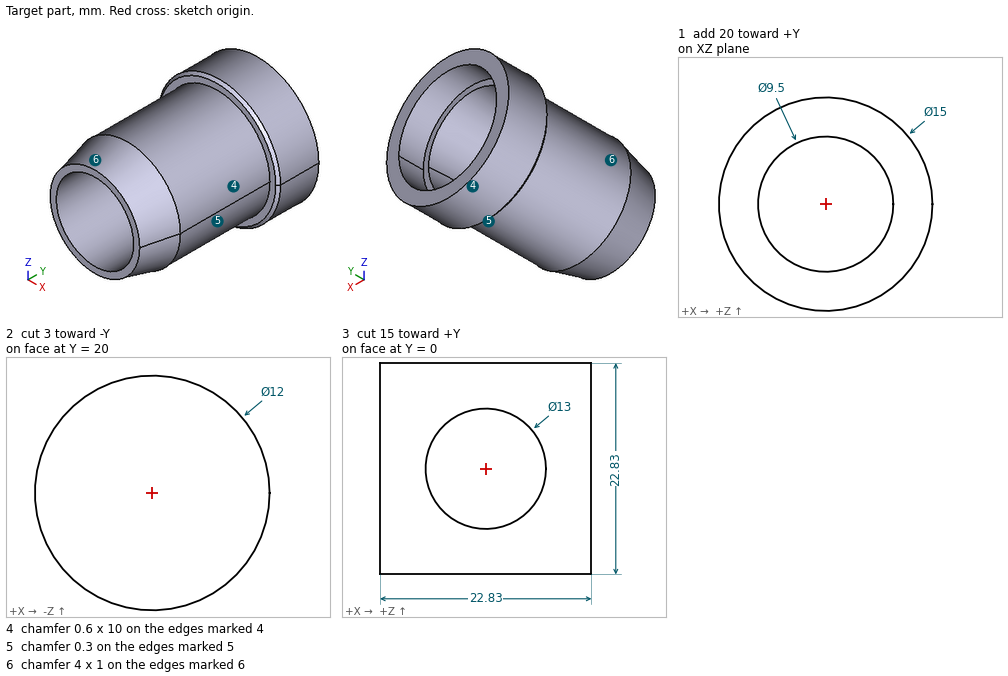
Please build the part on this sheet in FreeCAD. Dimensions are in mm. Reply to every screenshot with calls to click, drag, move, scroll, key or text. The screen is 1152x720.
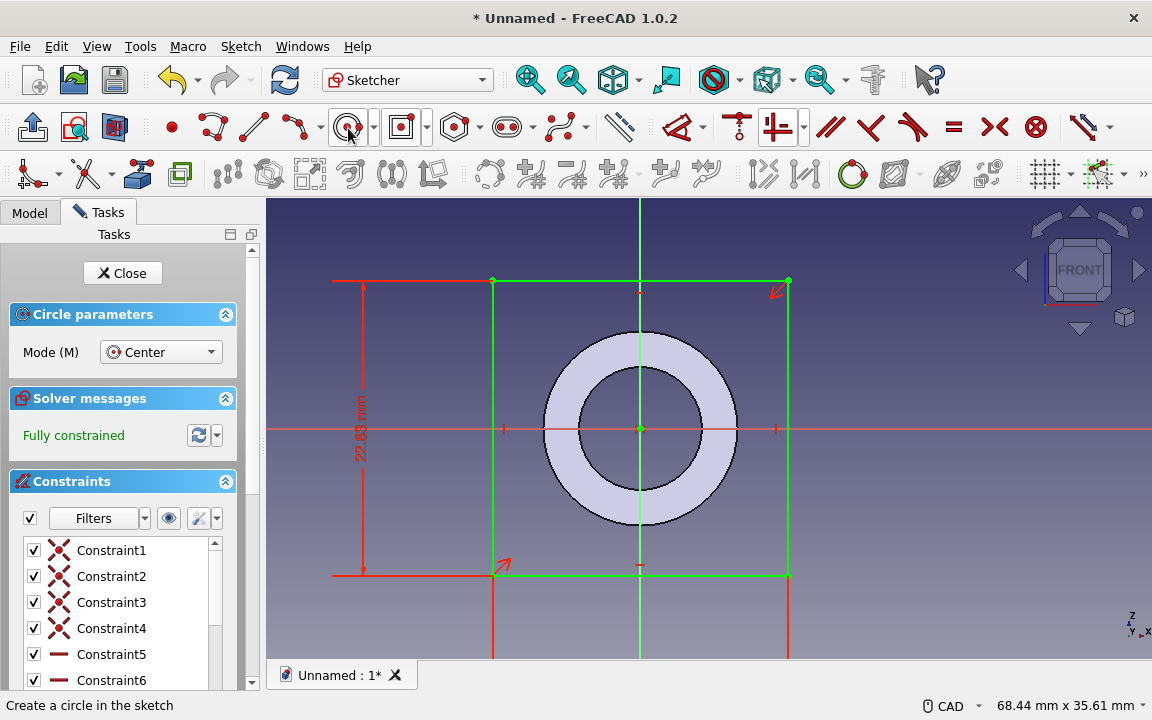
click(640, 429)
move(700, 369)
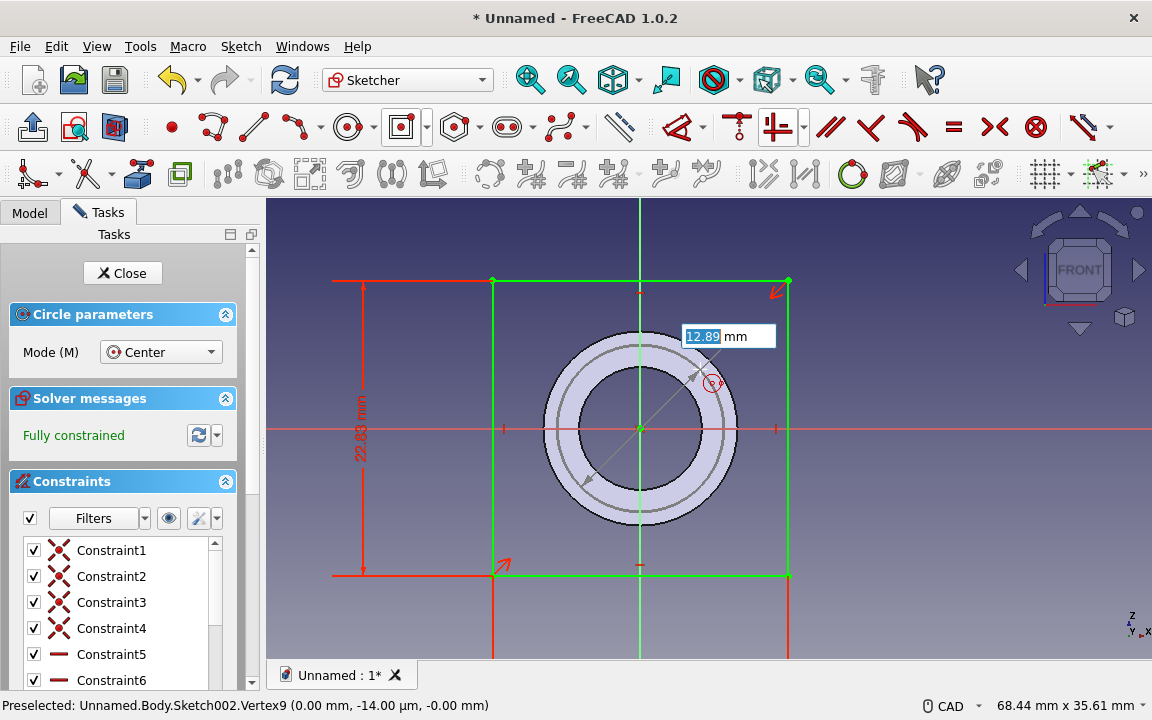
text(13)
key(Return)
key(Escape)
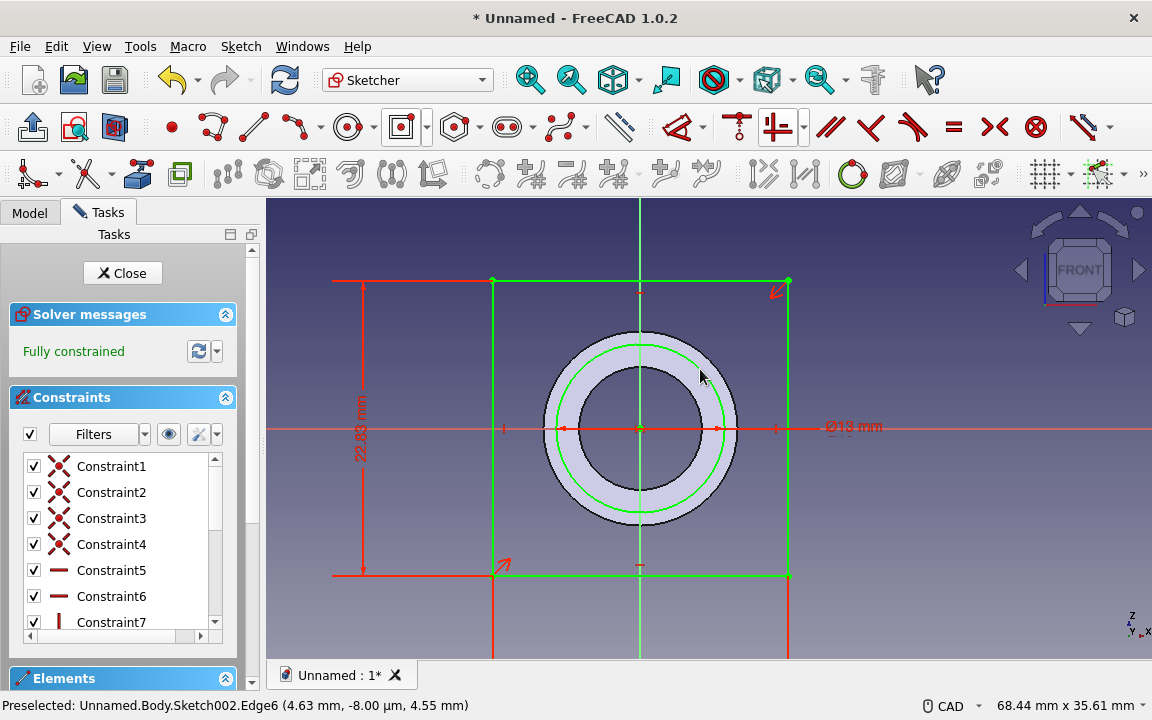
click(123, 273)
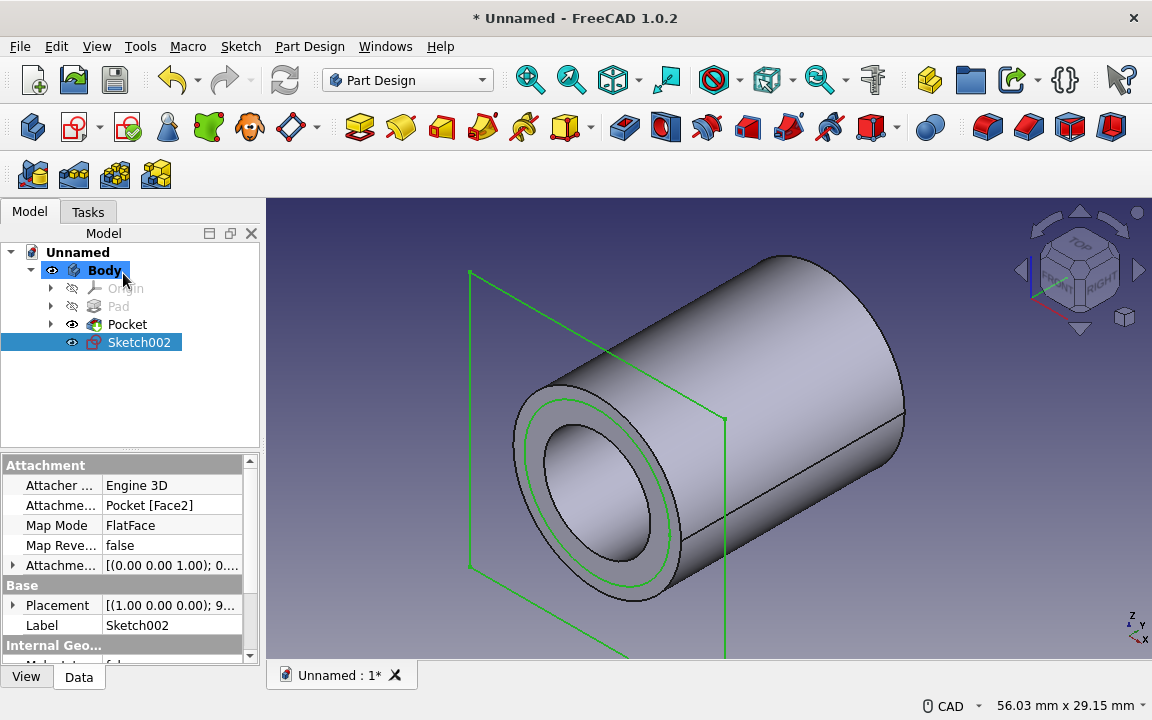
click(625, 128)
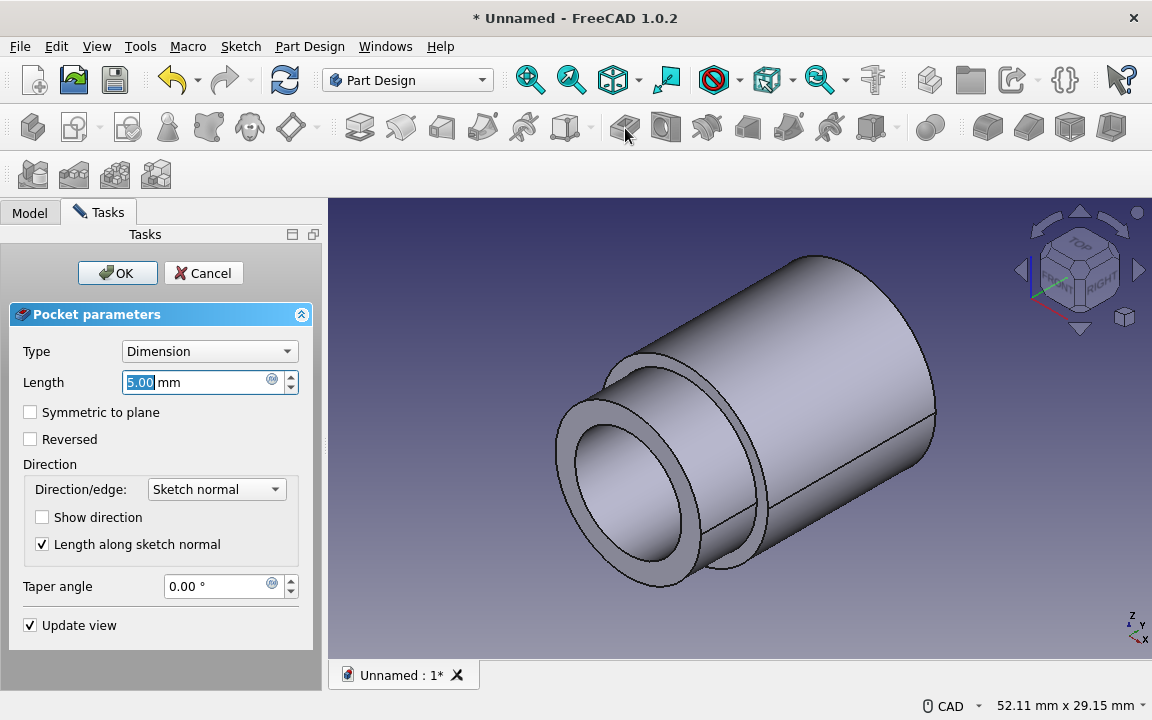
text(15)
key(Tab)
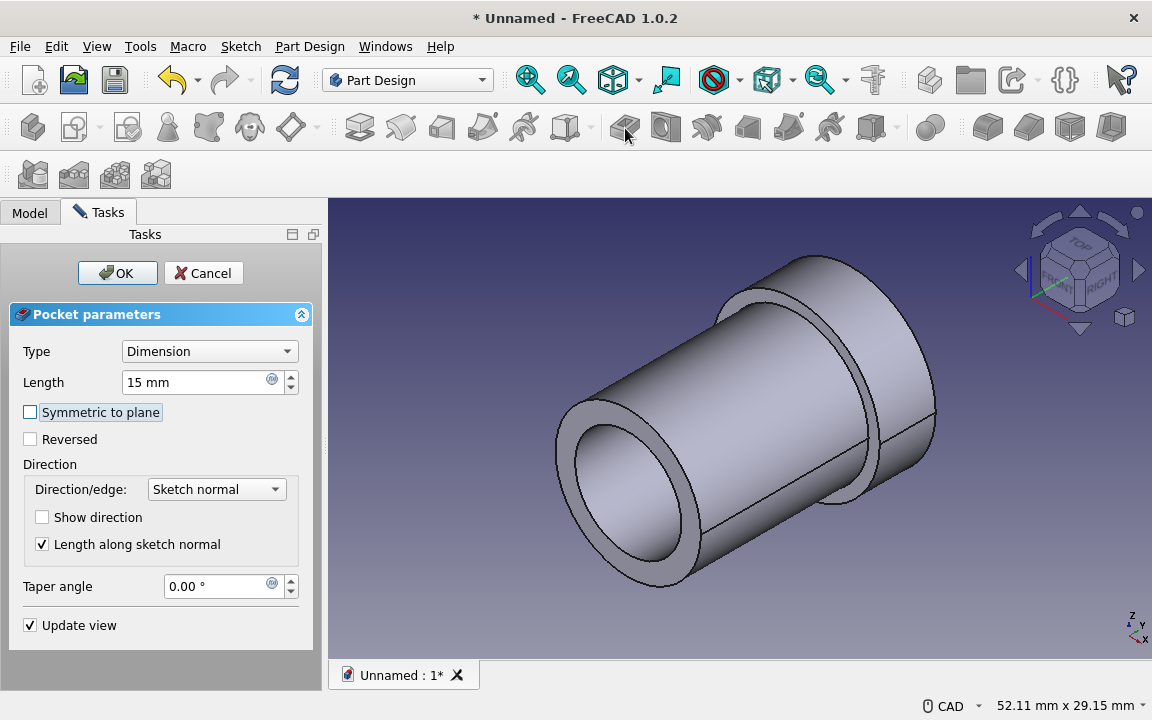
click(118, 273)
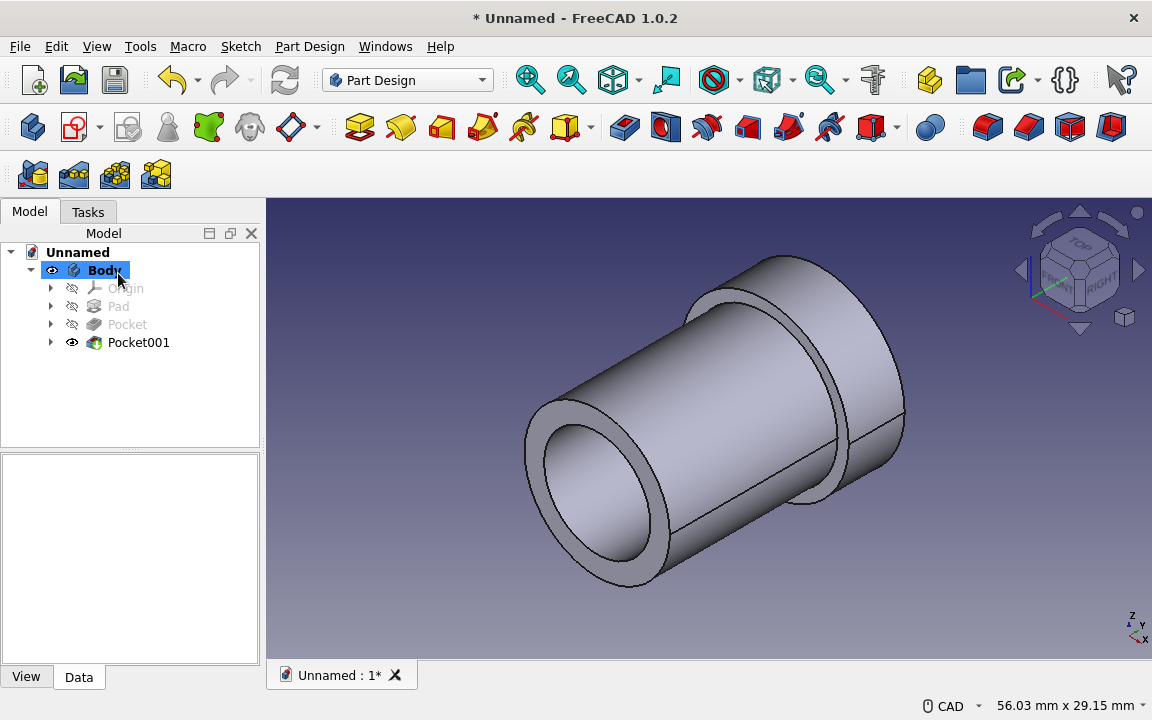
key(2)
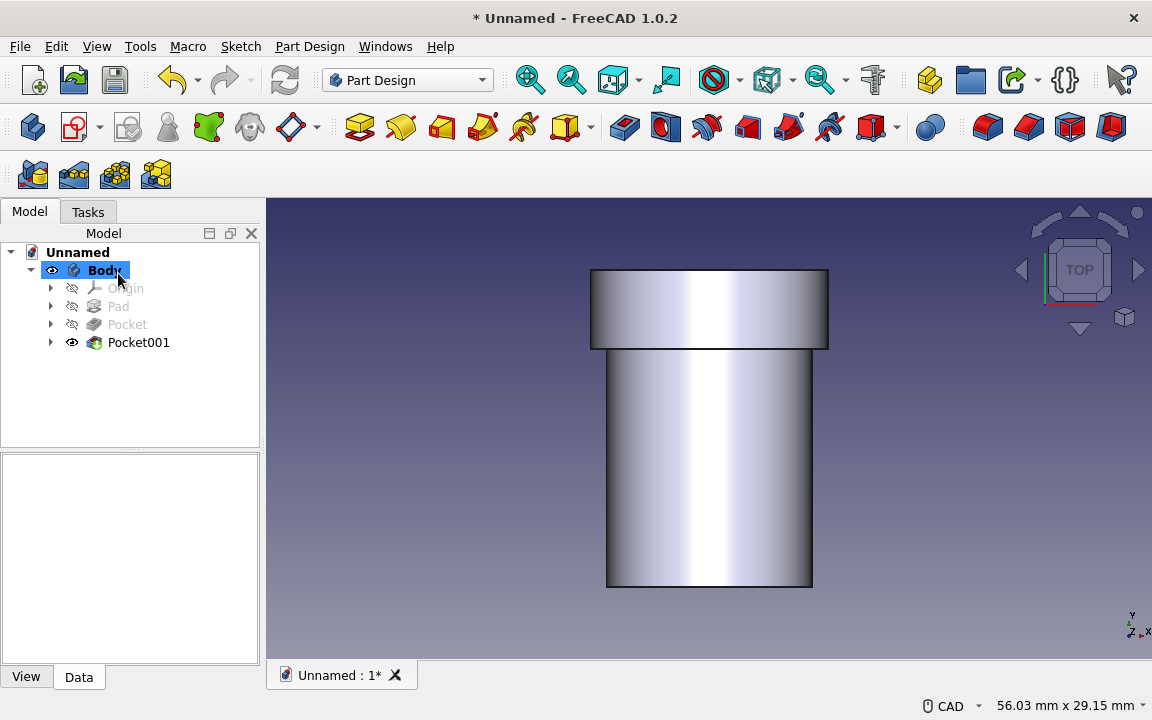
key(0)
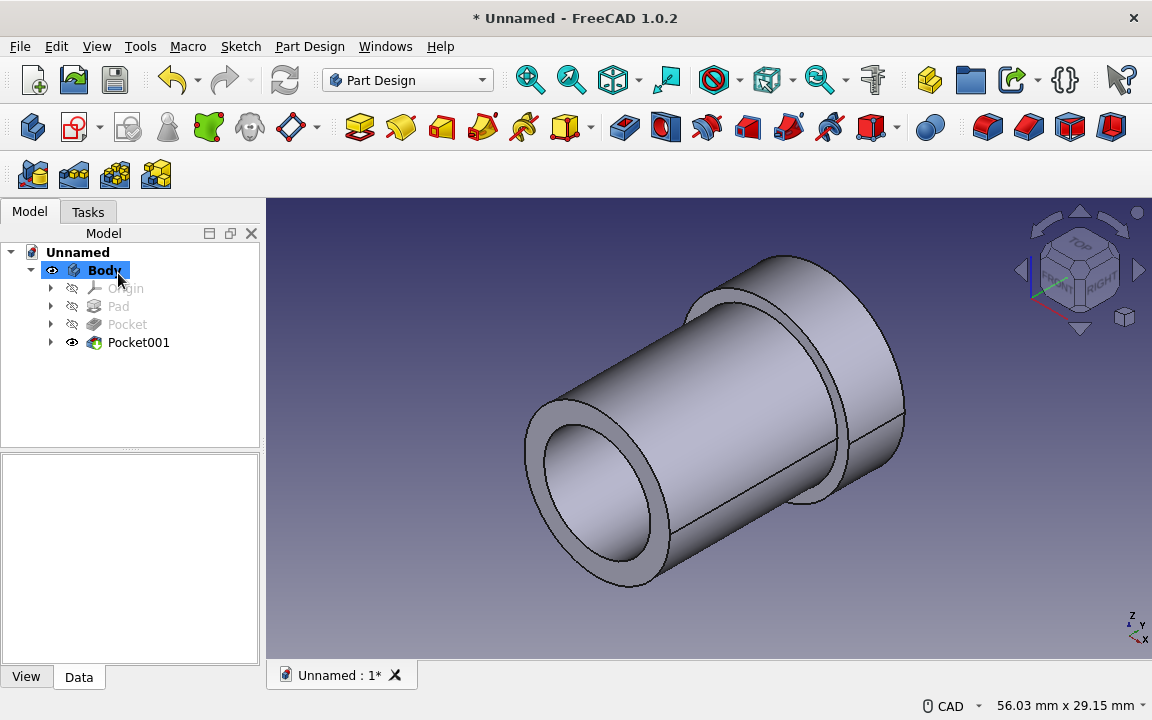
key(1)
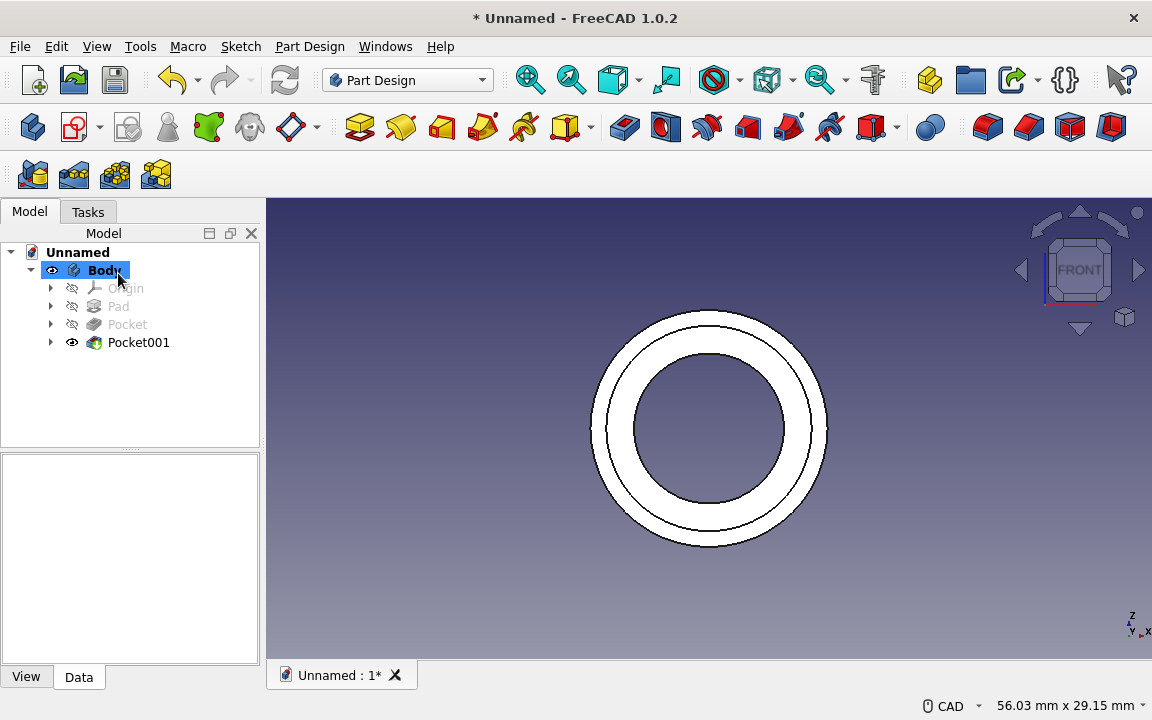
key(3)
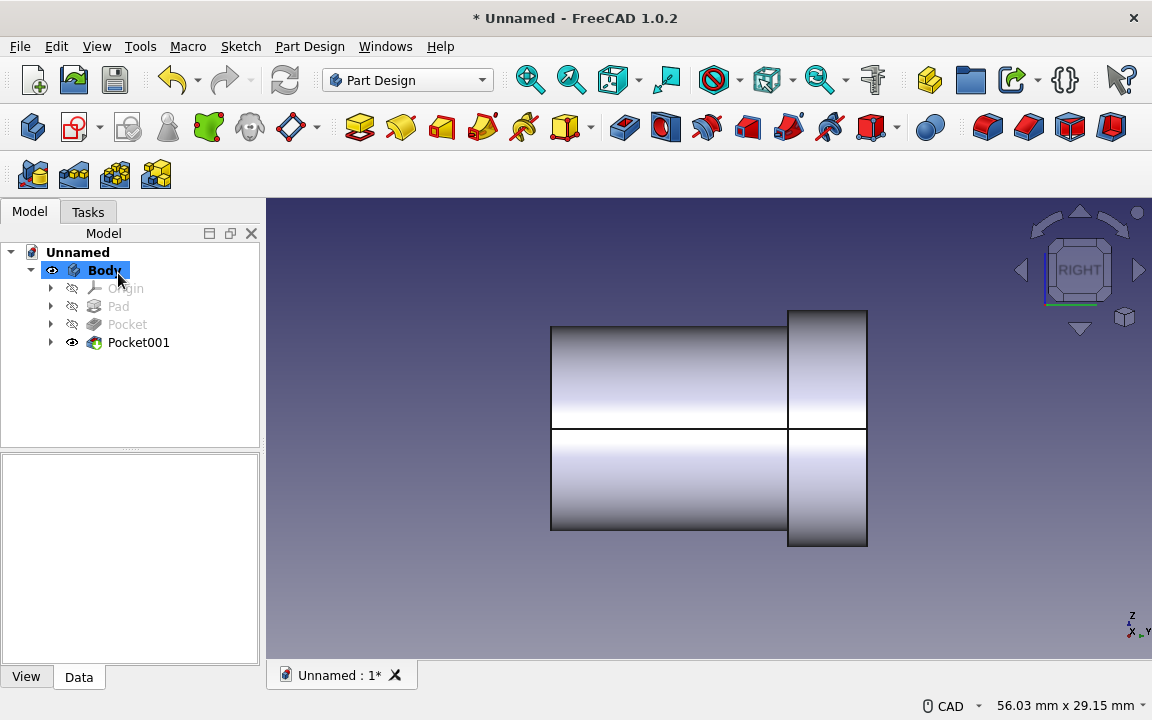
key(5)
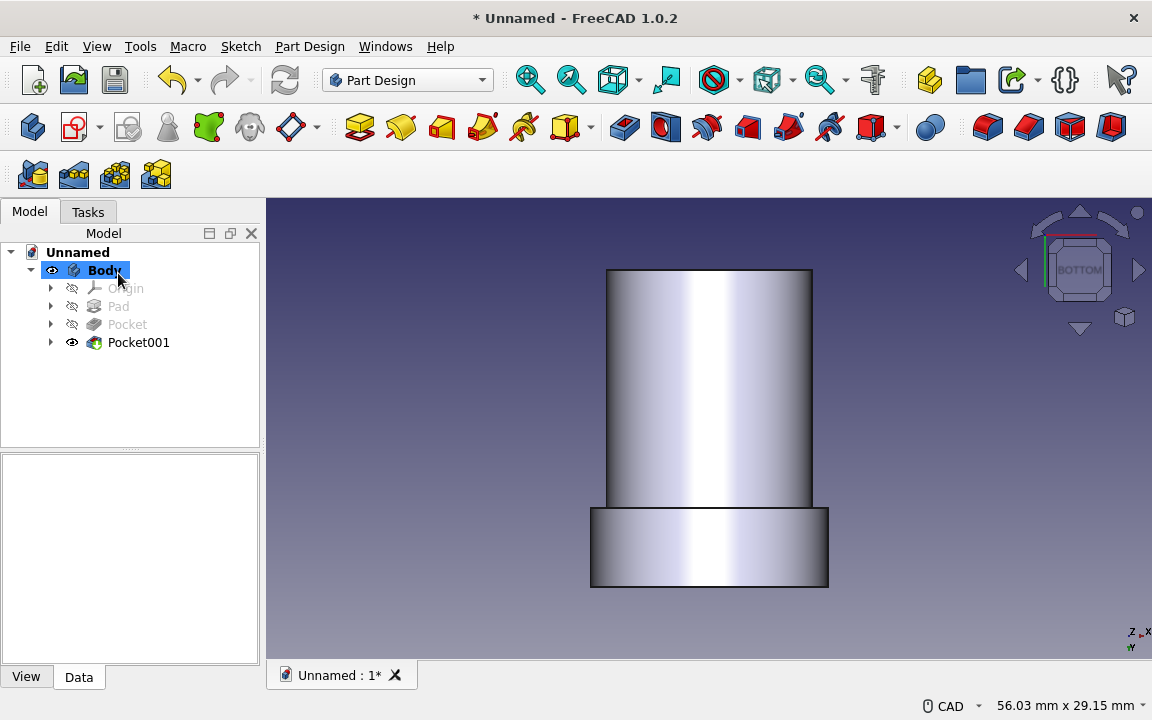
key(4)